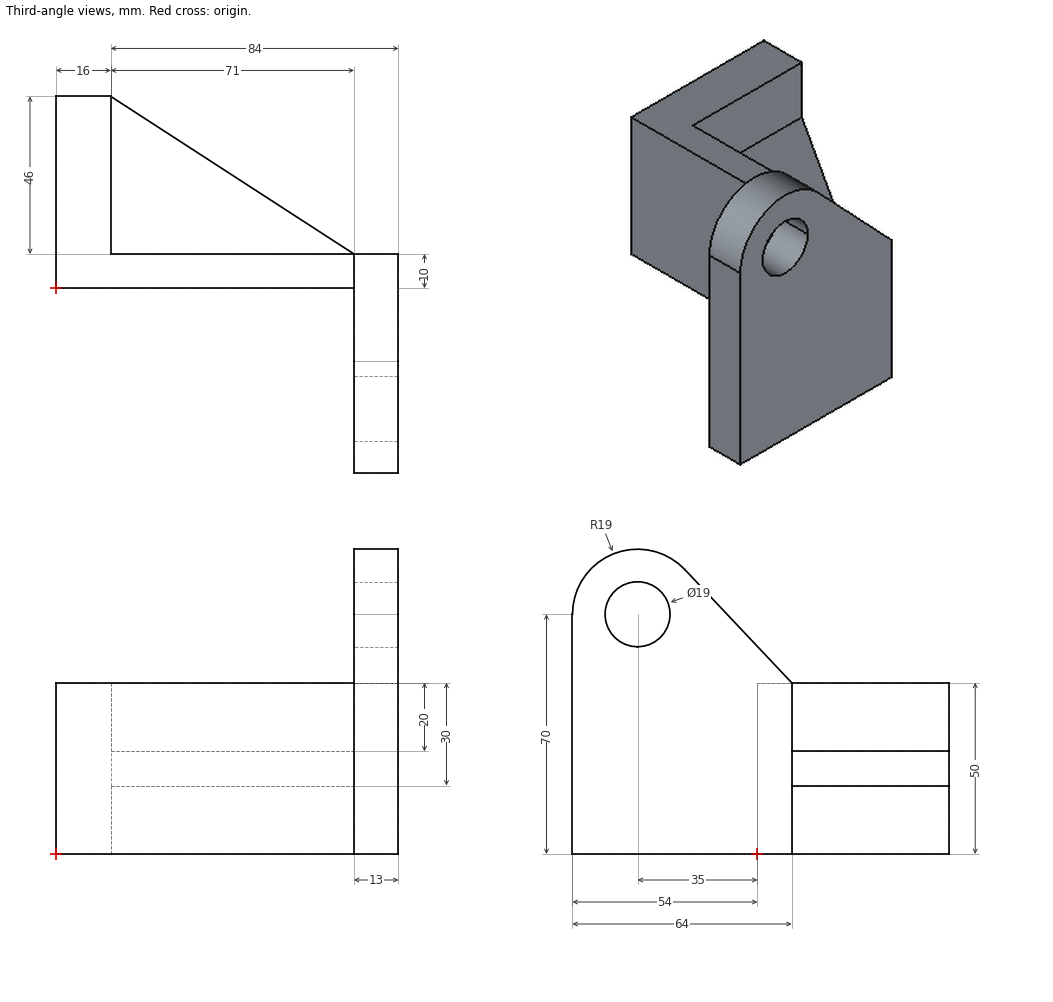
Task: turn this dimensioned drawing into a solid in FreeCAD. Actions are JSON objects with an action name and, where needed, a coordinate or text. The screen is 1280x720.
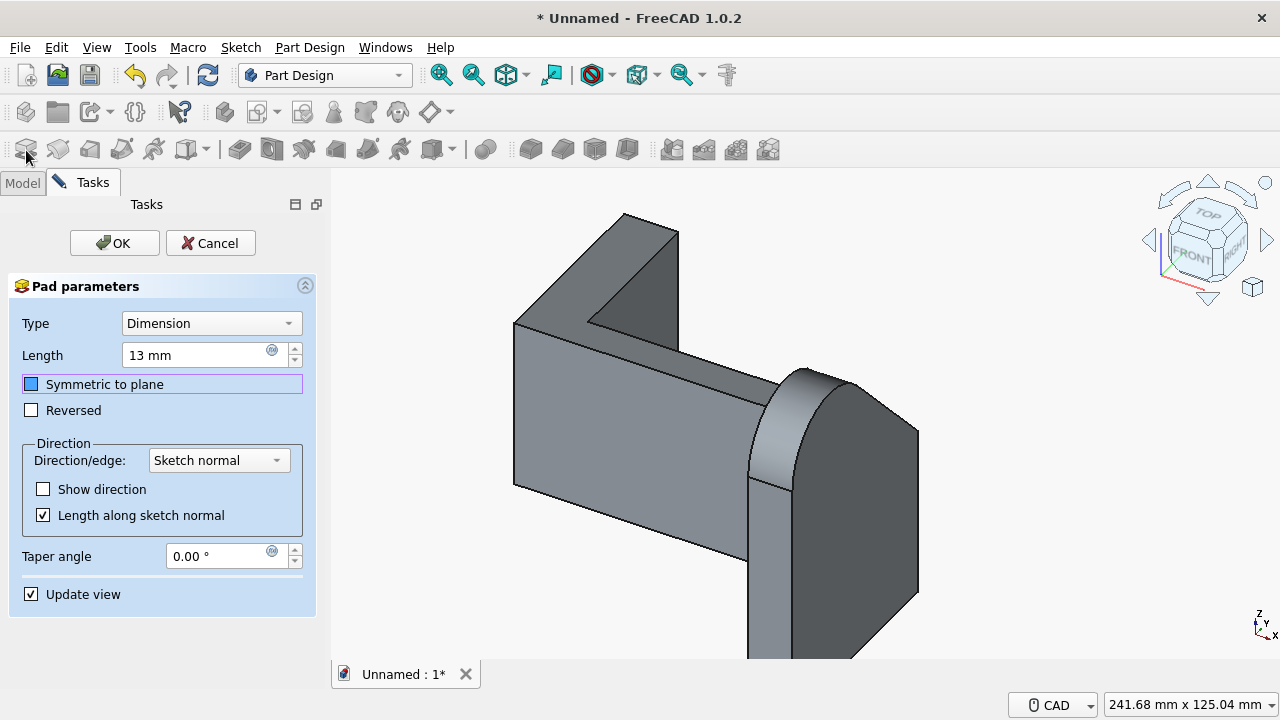
{"action": "left_click", "coordinate": [30, 410]}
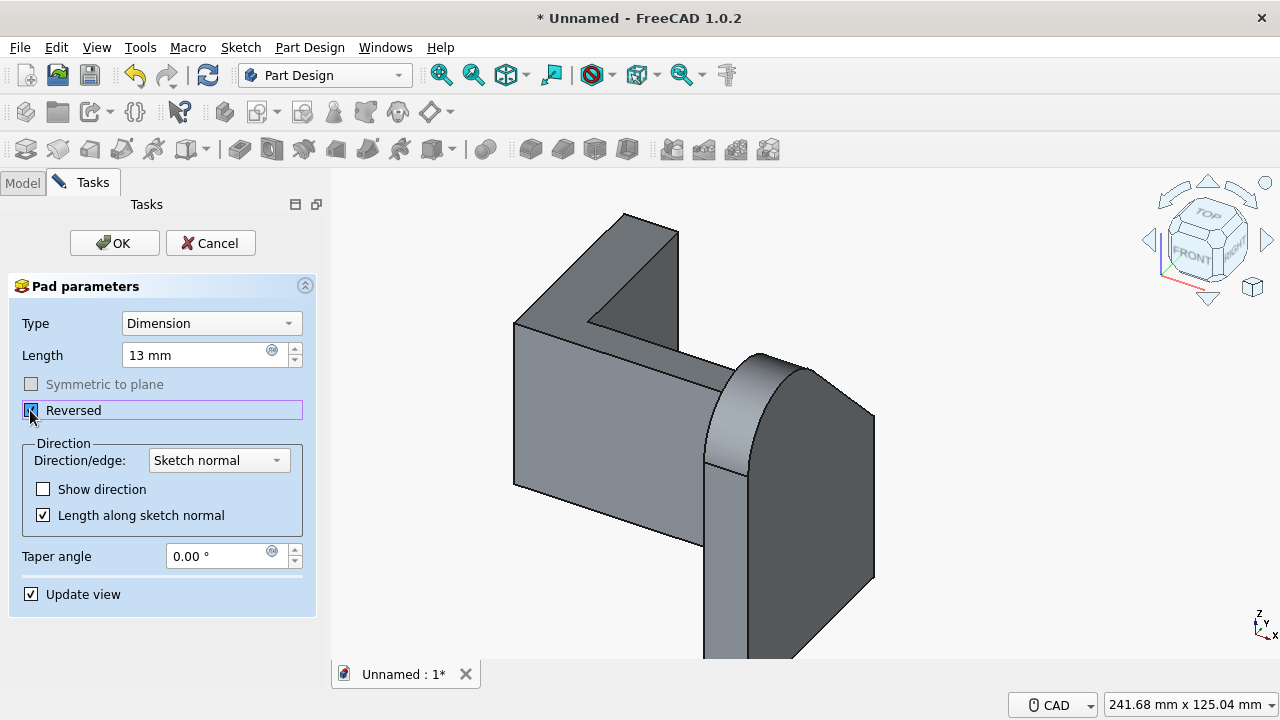
{"action": "left_click", "coordinate": [115, 243]}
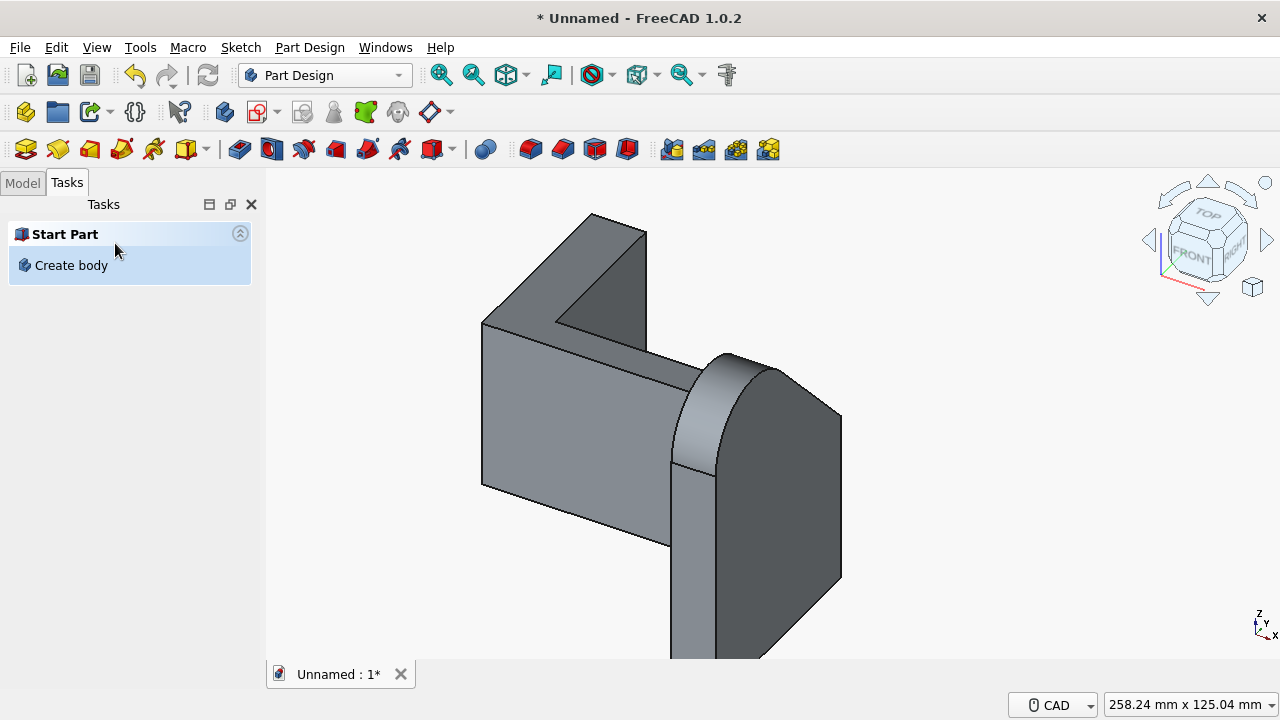
{"action": "left_click", "coordinate": [442, 76]}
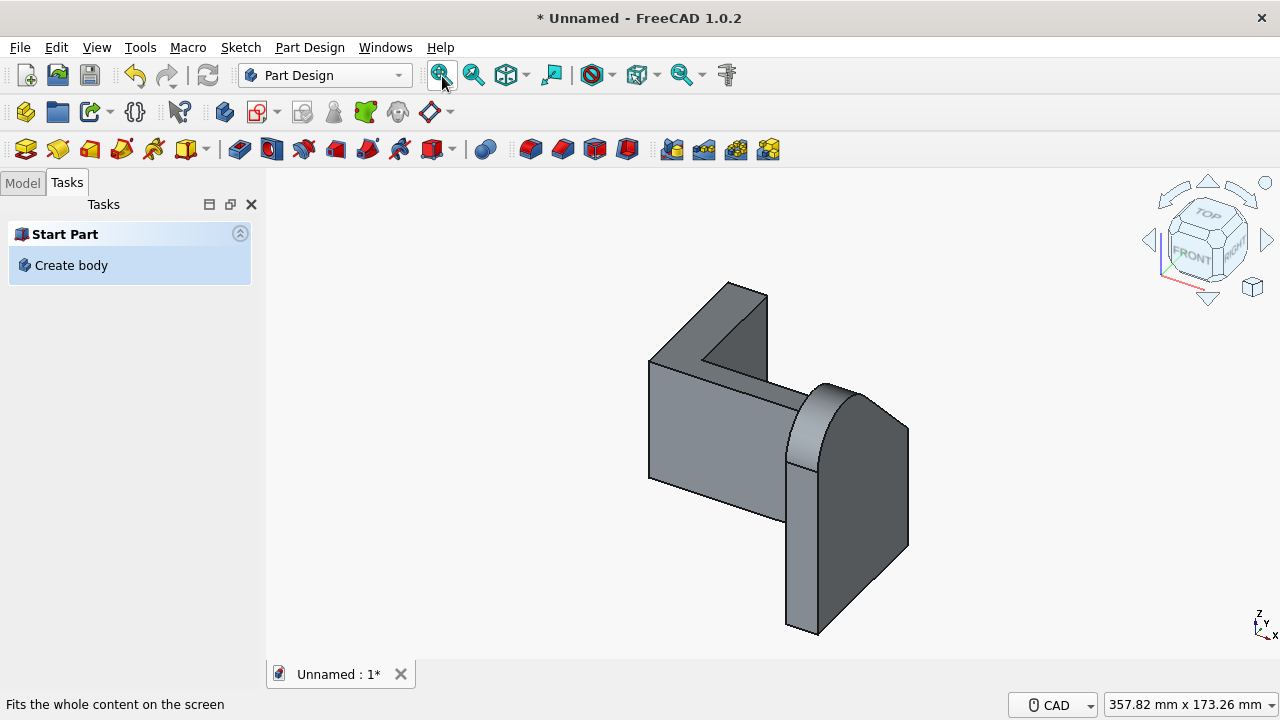
{"action": "left_click", "coordinate": [863, 515]}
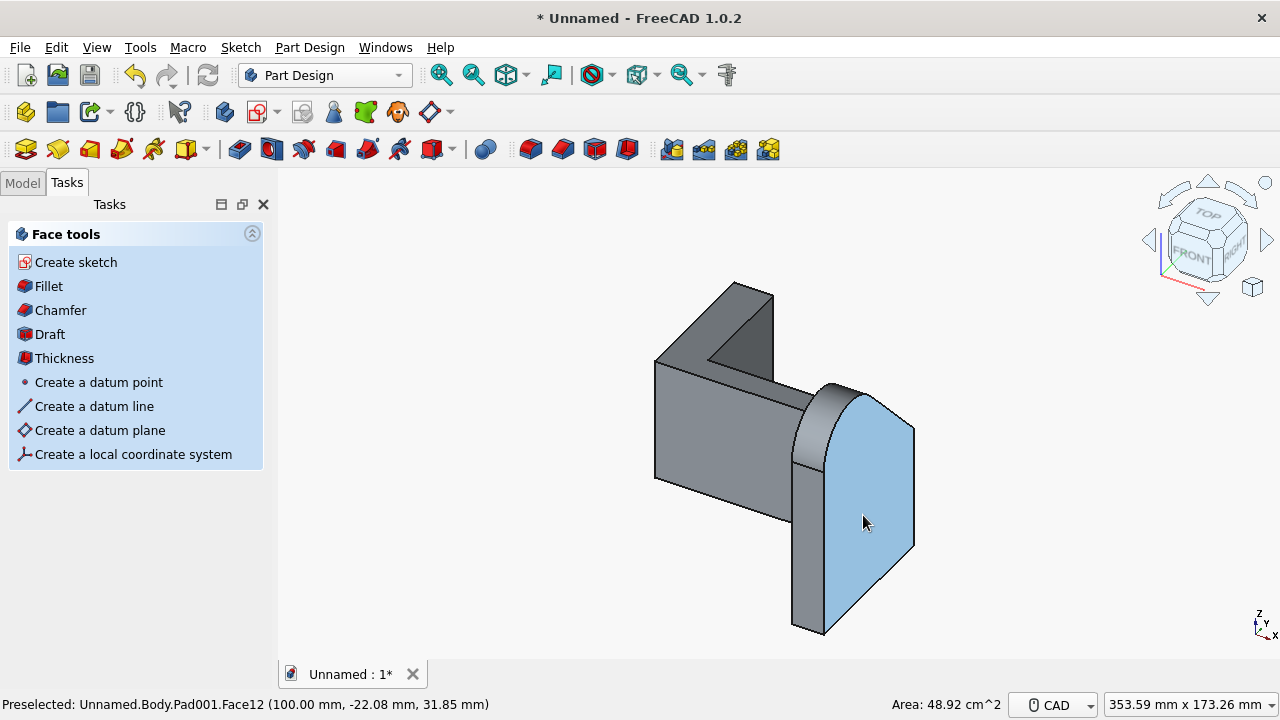
{"action": "left_click", "coordinate": [258, 112]}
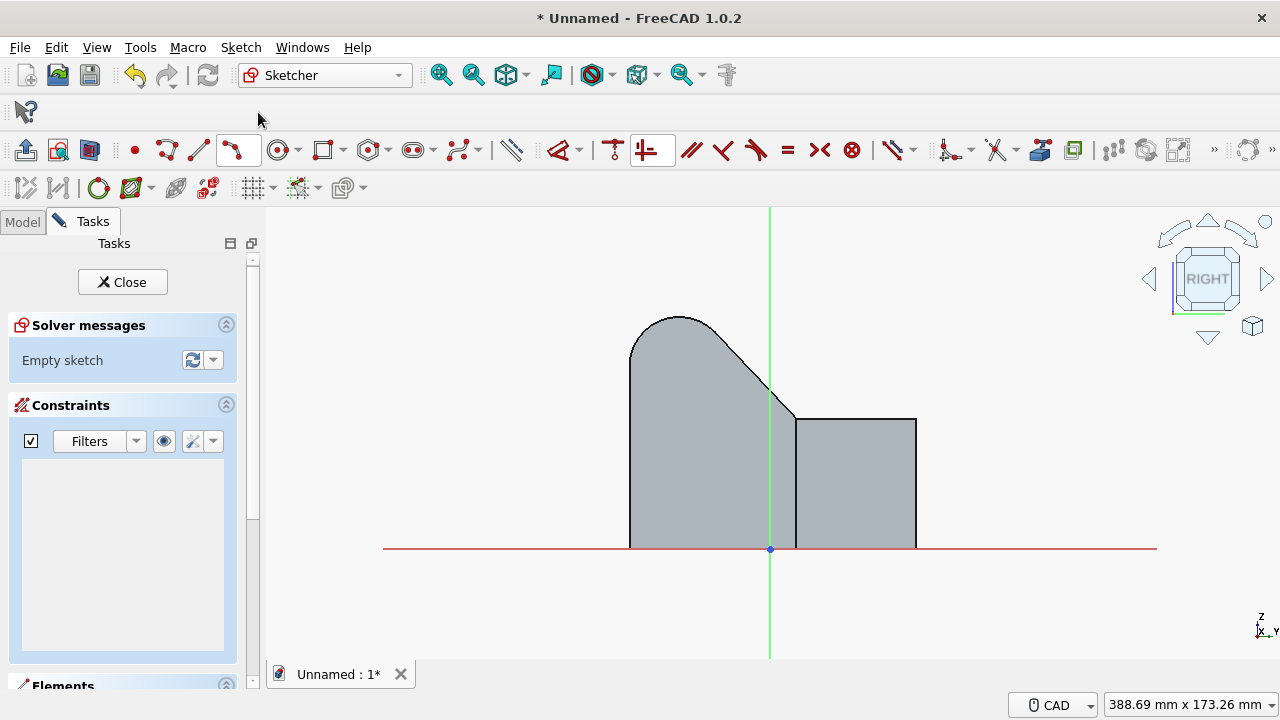
{"action": "scroll", "coordinate": [674, 353], "scroll_direction": "up", "scroll_amount": 9}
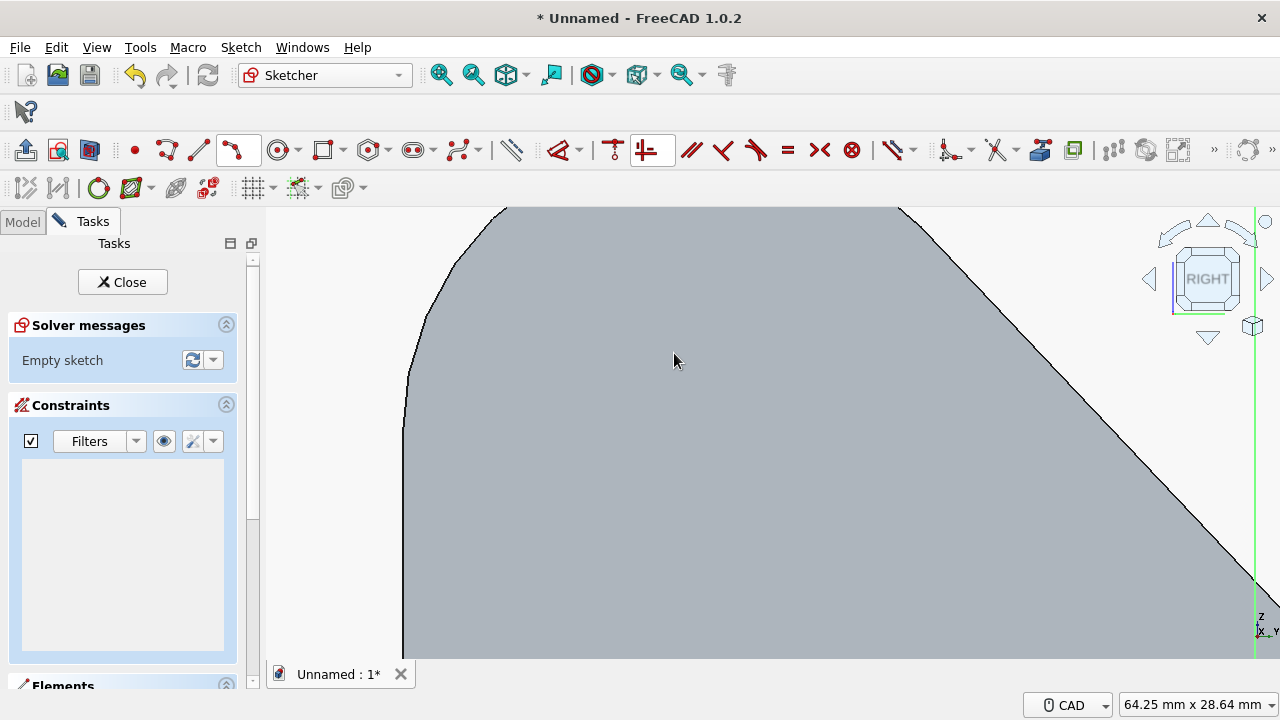
{"action": "key", "text": "g c"}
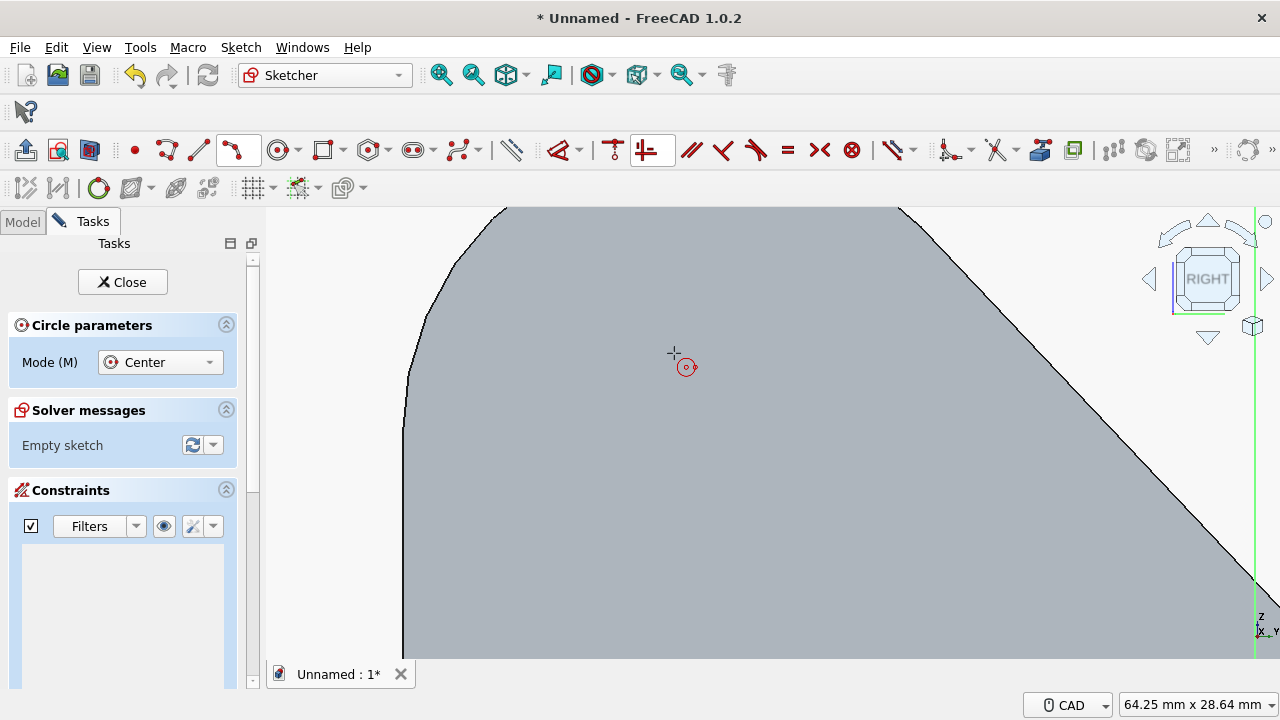
{"action": "left_click", "coordinate": [703, 433]}
{"action": "left_click", "coordinate": [809, 327]}
{"action": "key", "text": "Escape"}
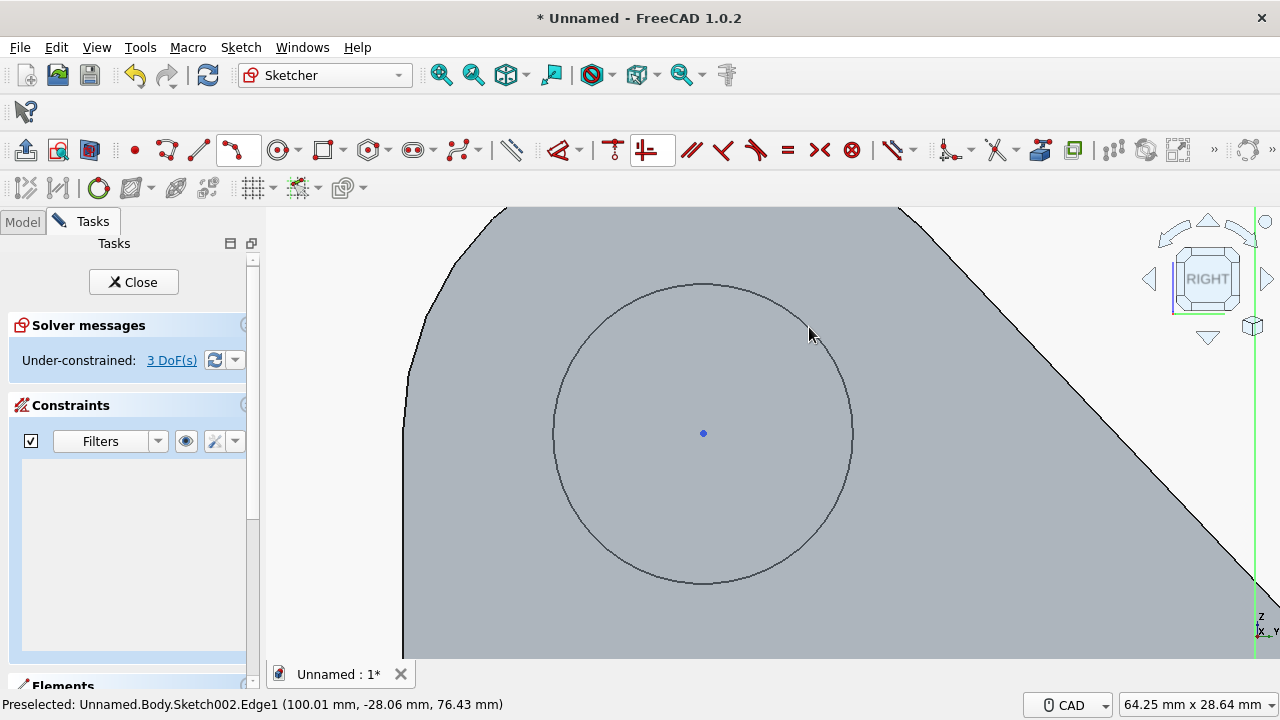
{"action": "key", "text": "d"}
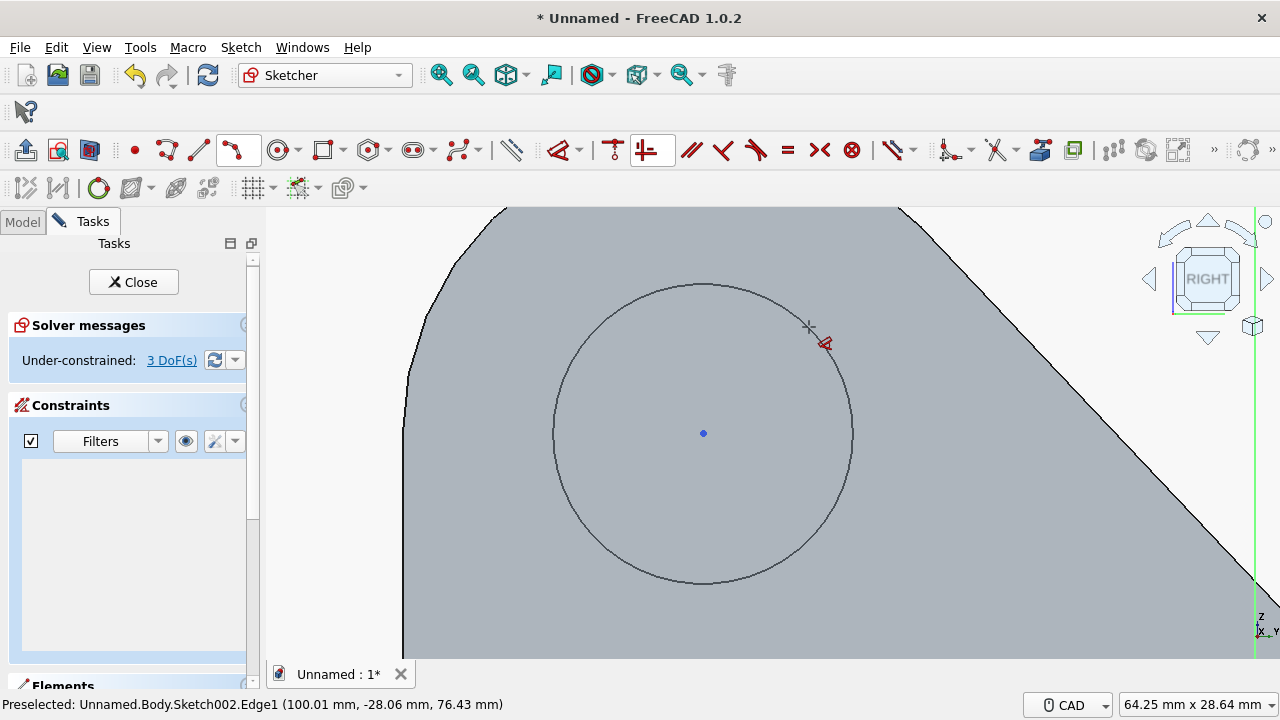
{"action": "left_click", "coordinate": [809, 328]}
{"action": "left_click", "coordinate": [832, 305]}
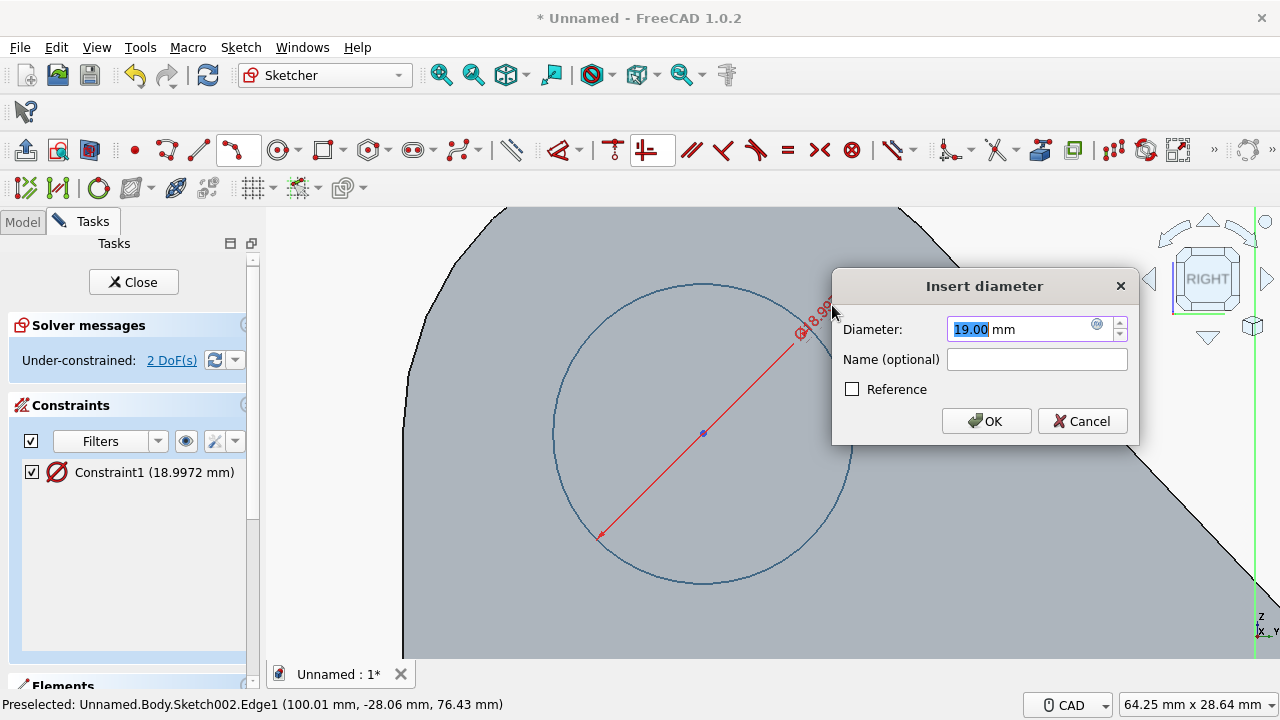
{"action": "type", "text": "19"}
{"action": "key", "text": "Return"}